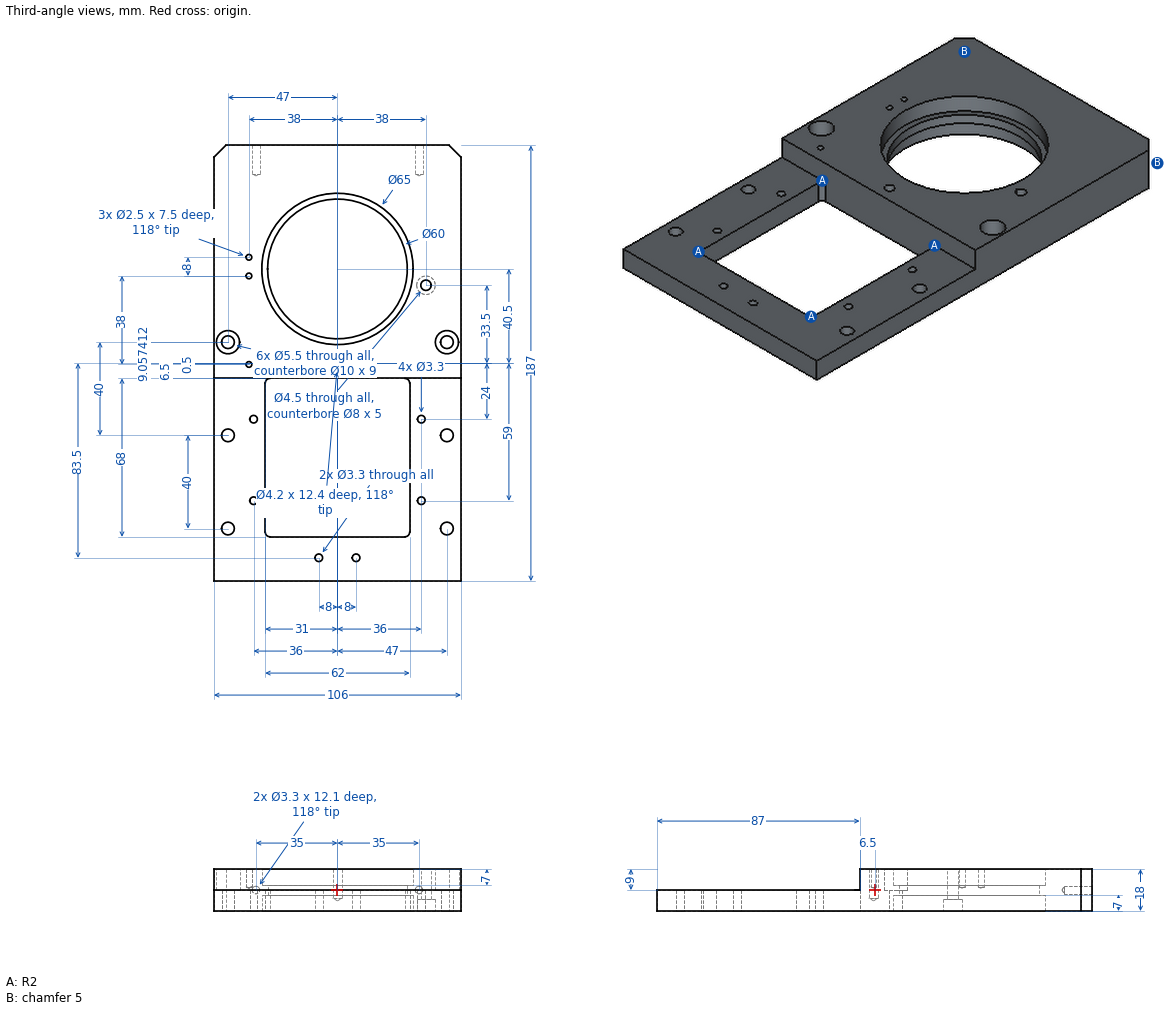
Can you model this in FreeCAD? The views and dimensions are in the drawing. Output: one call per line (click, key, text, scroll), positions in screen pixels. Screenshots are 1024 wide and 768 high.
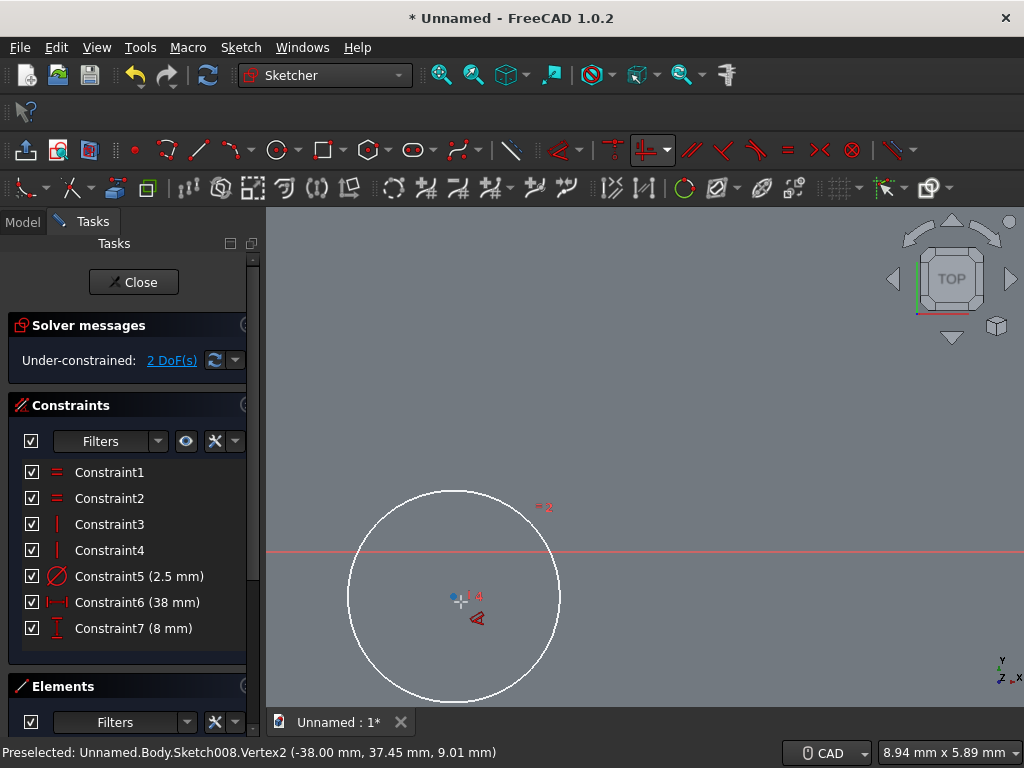
click(454, 597)
click(420, 574)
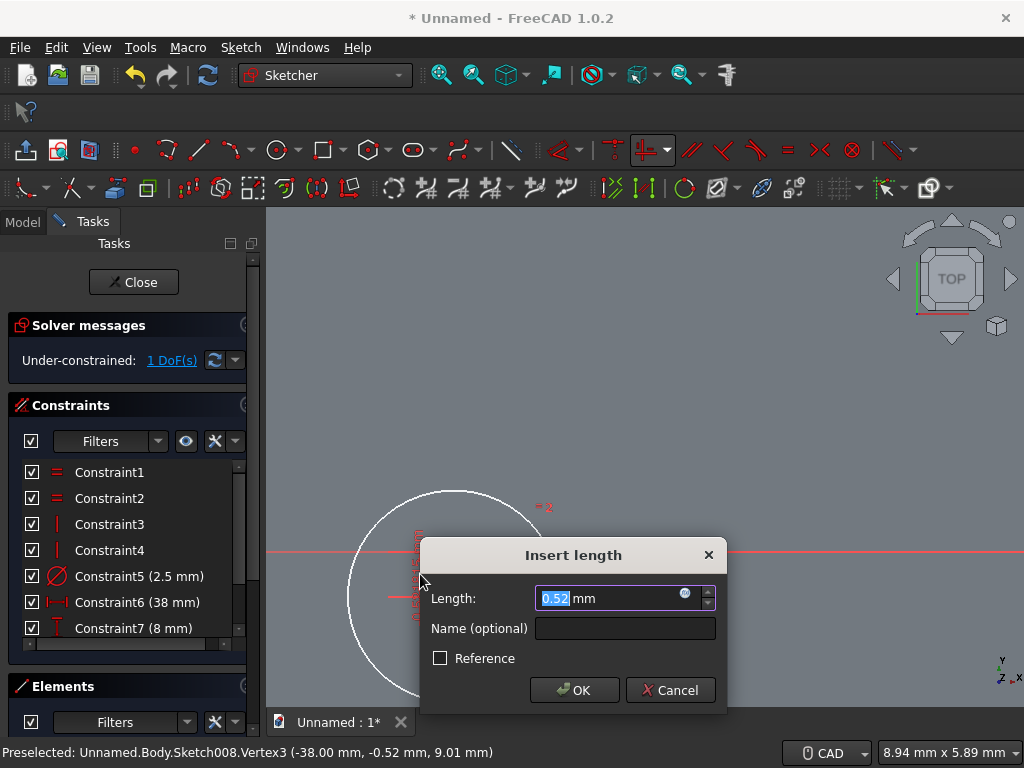
text(0.5)
key(Return)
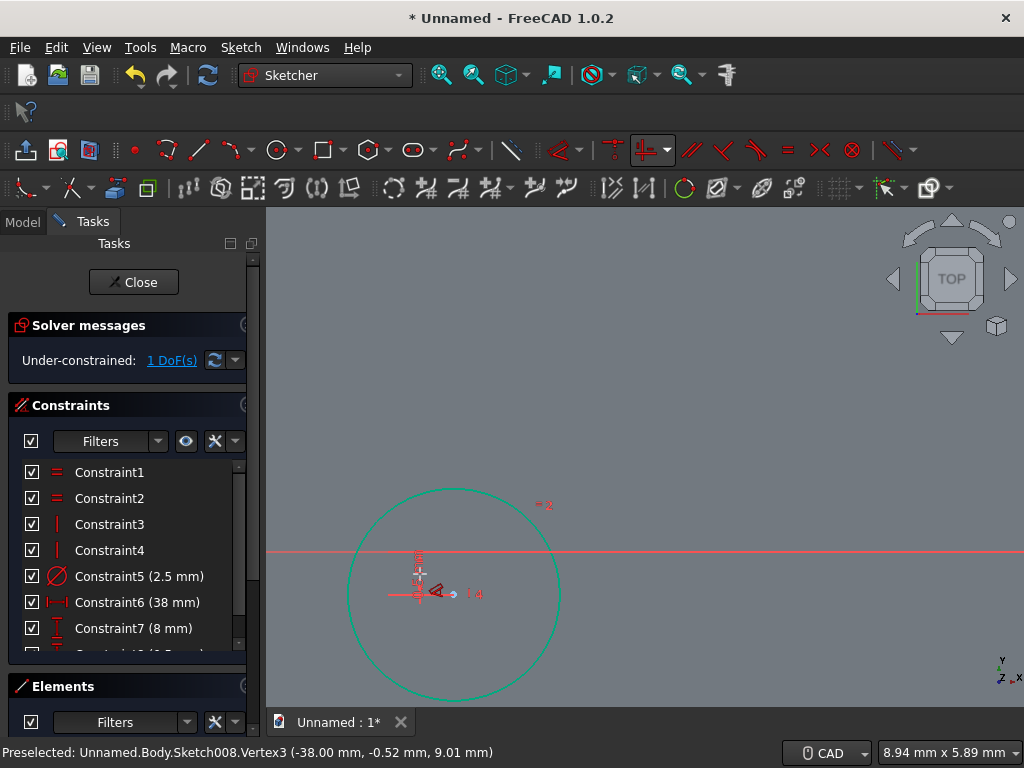
scroll(461, 602, down, 13)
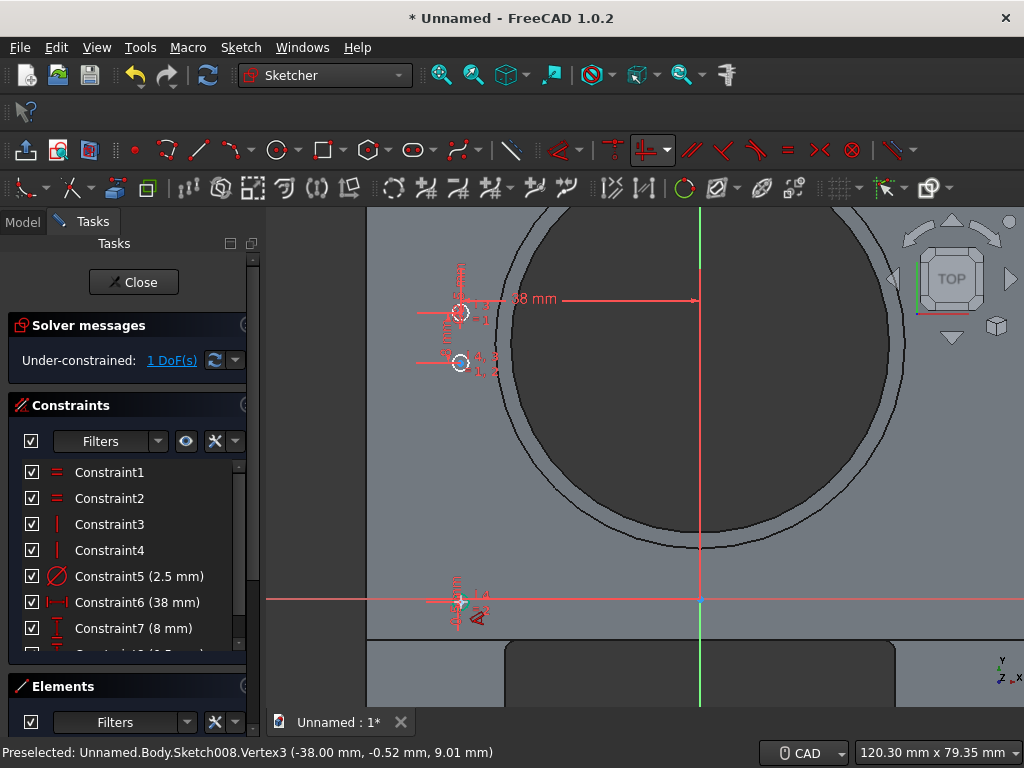
click(461, 363)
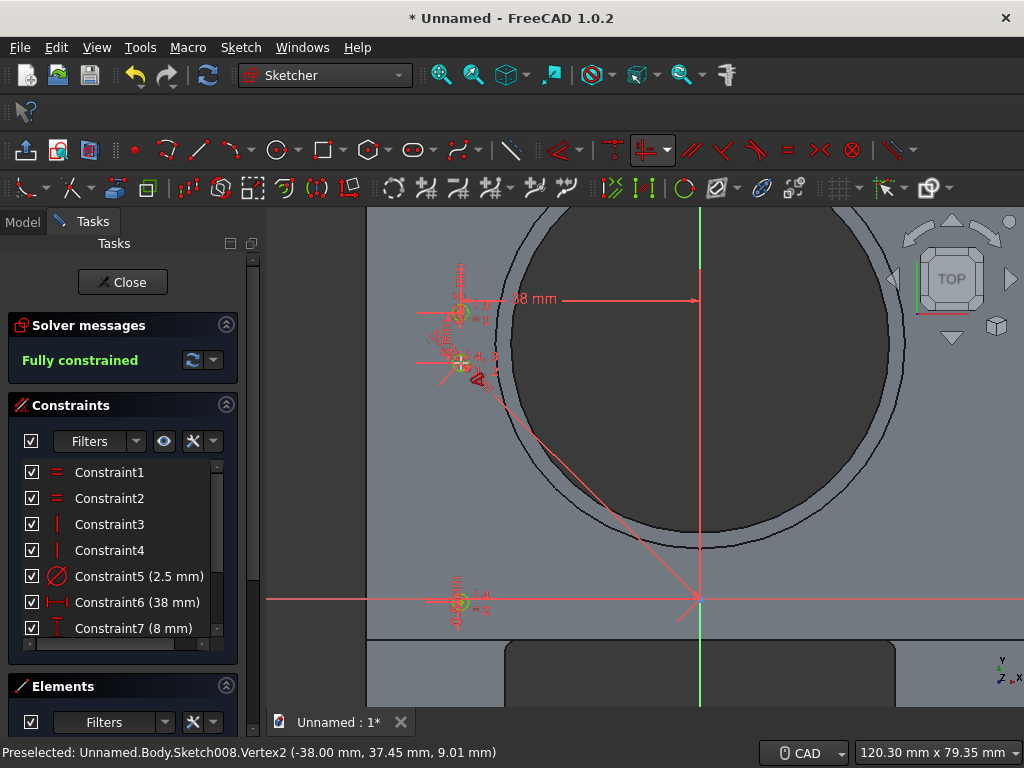
click(461, 602)
click(427, 483)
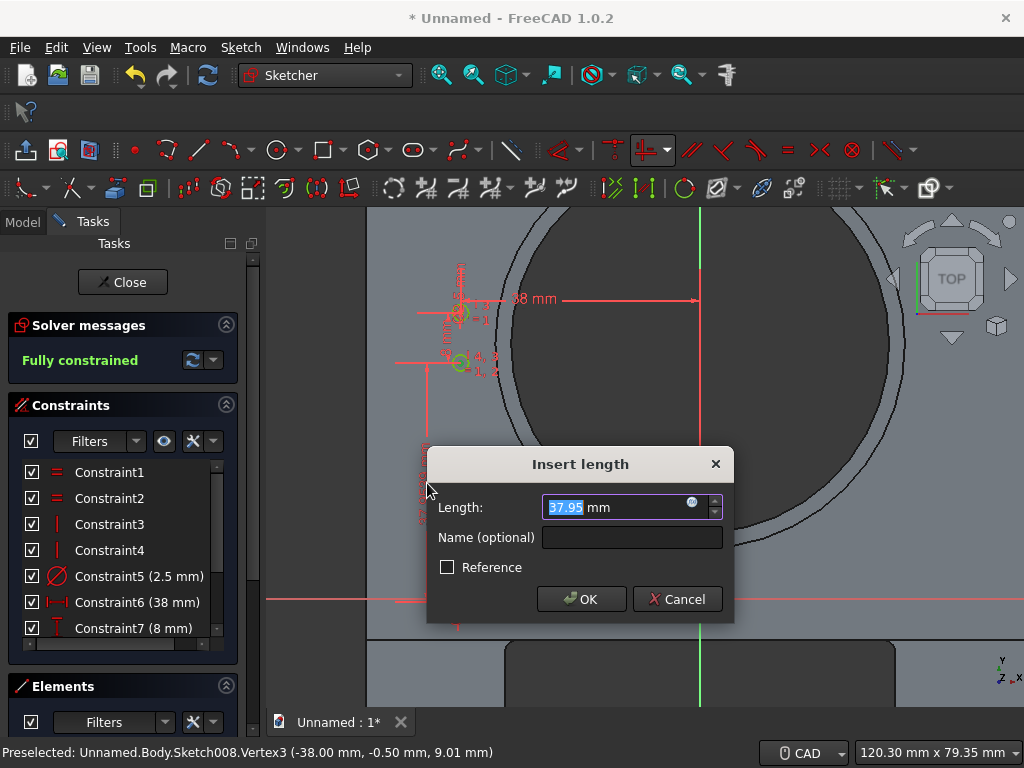
text(38)
key(Return)
key(Escape)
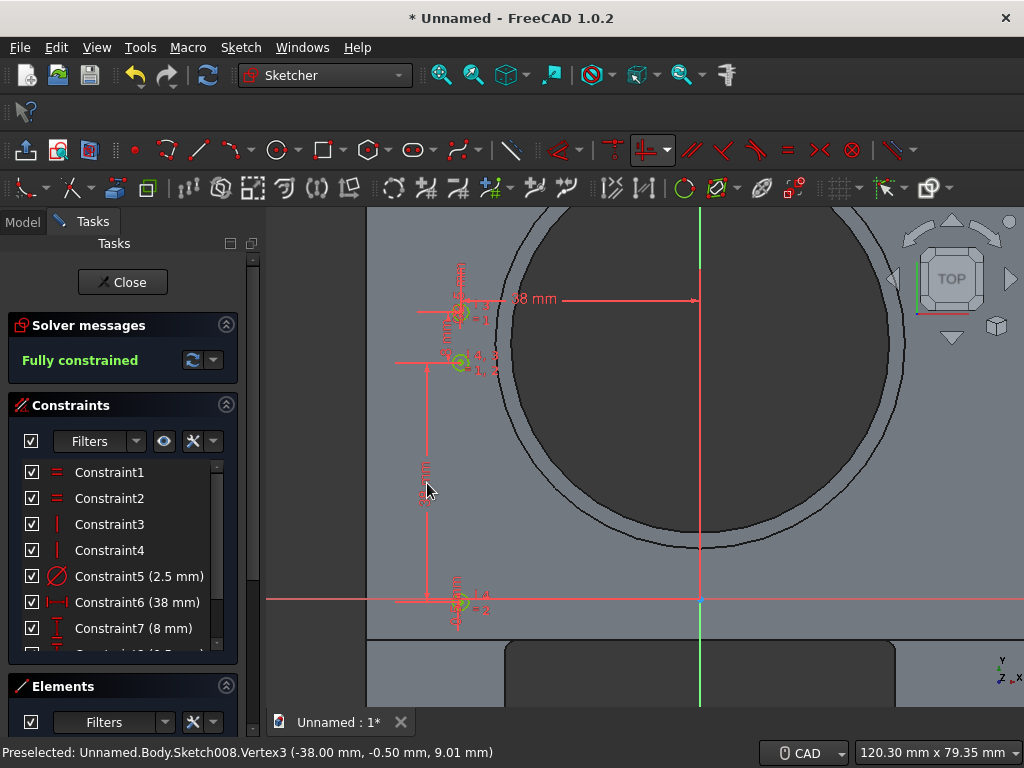
click(123, 282)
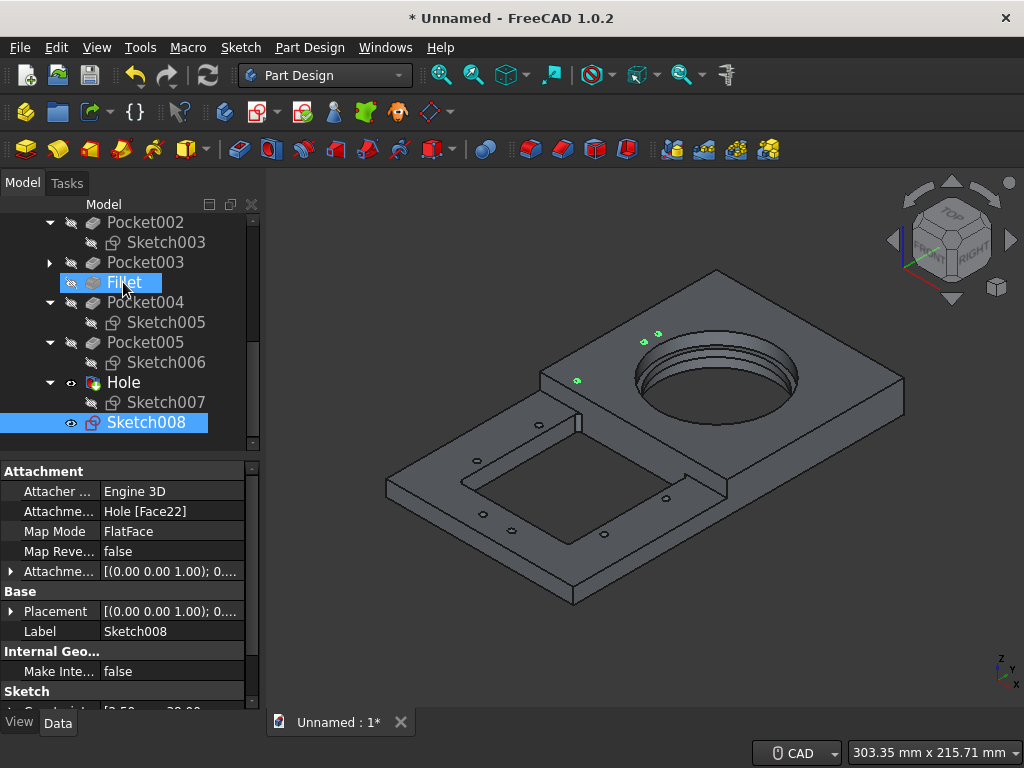
click(272, 150)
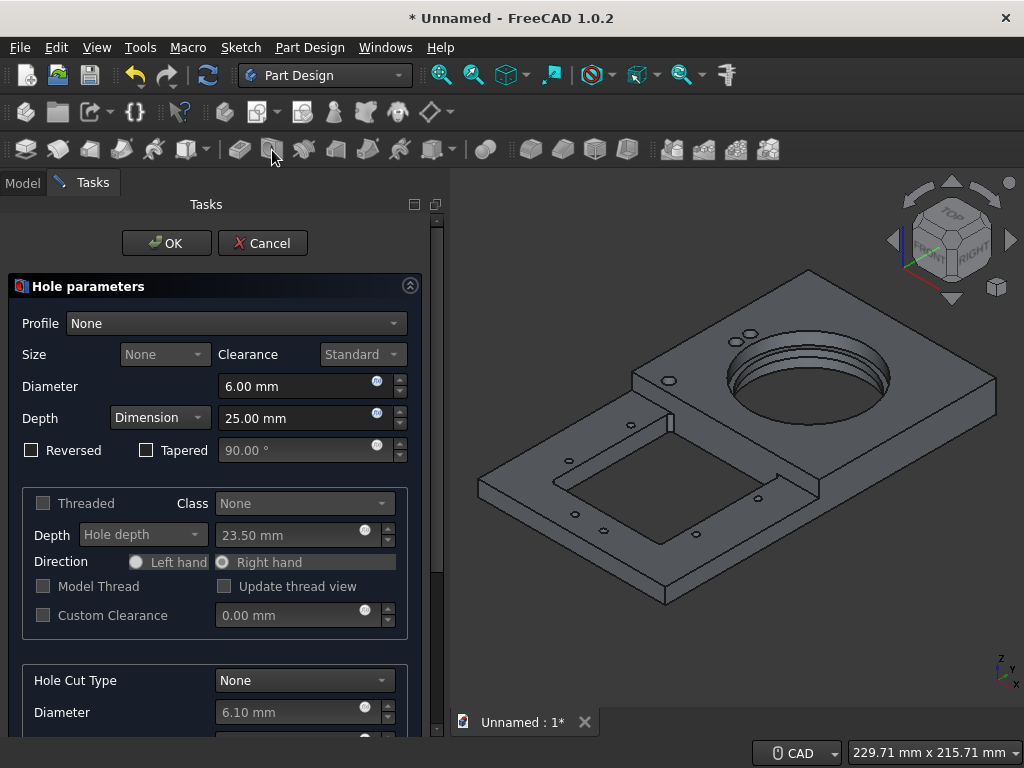
triple_click(305, 386)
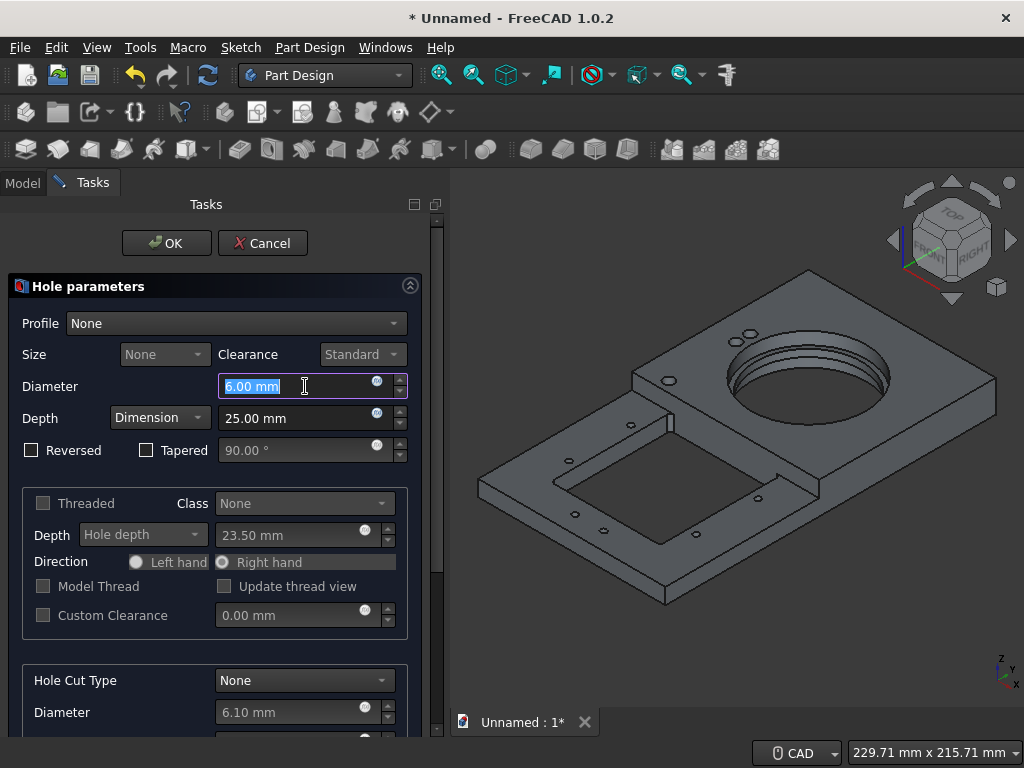
text(2.5)
key(Tab)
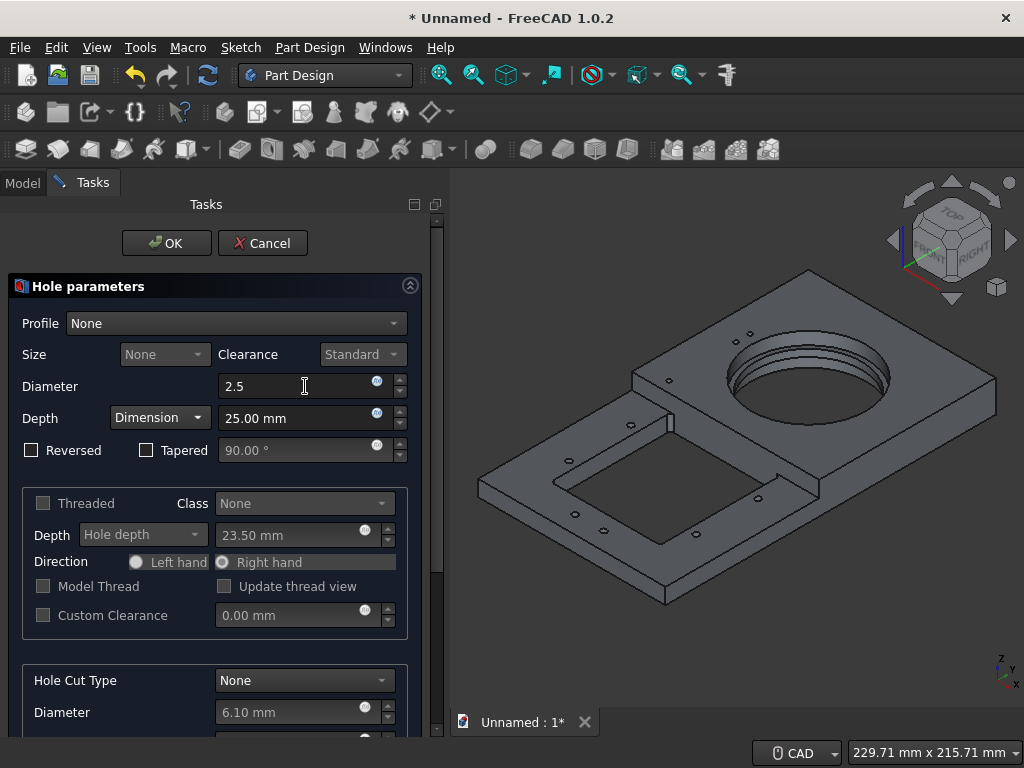
triple_click(305, 418)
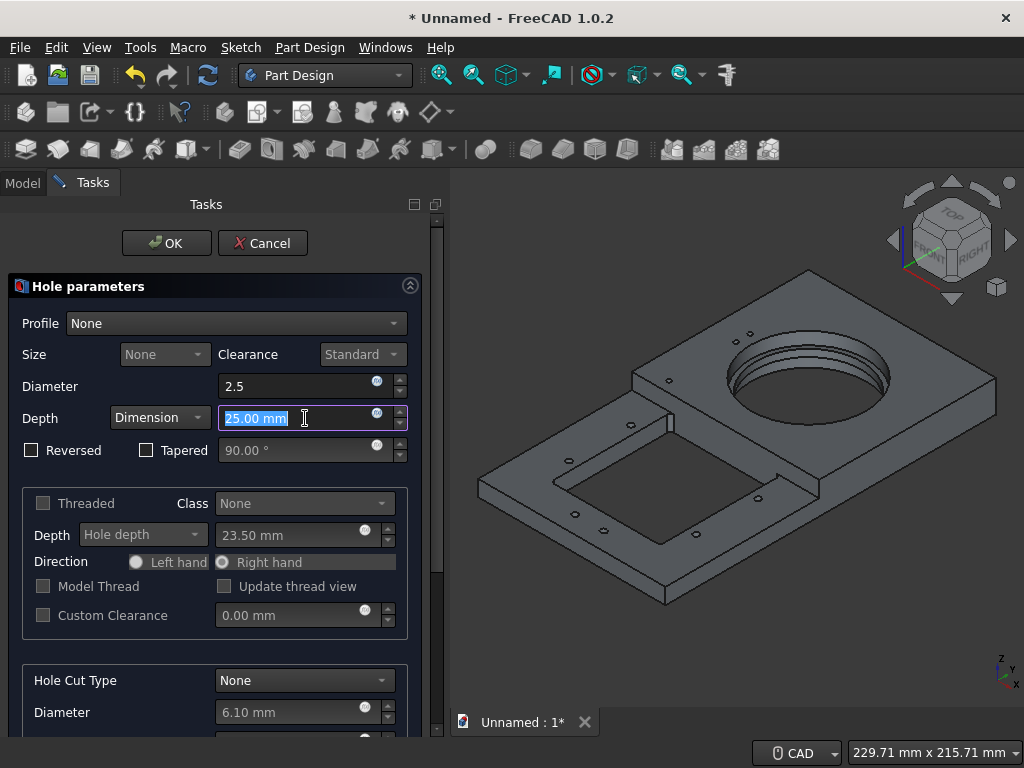
text(7.5)
key(Tab)